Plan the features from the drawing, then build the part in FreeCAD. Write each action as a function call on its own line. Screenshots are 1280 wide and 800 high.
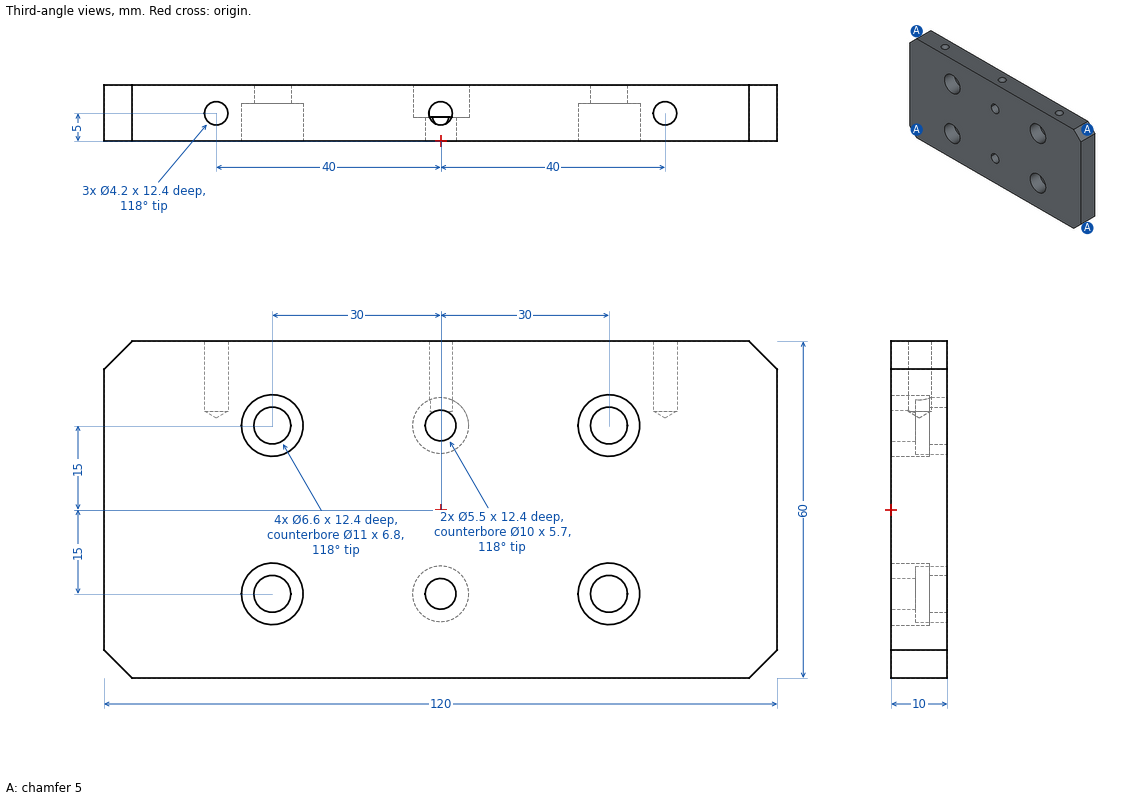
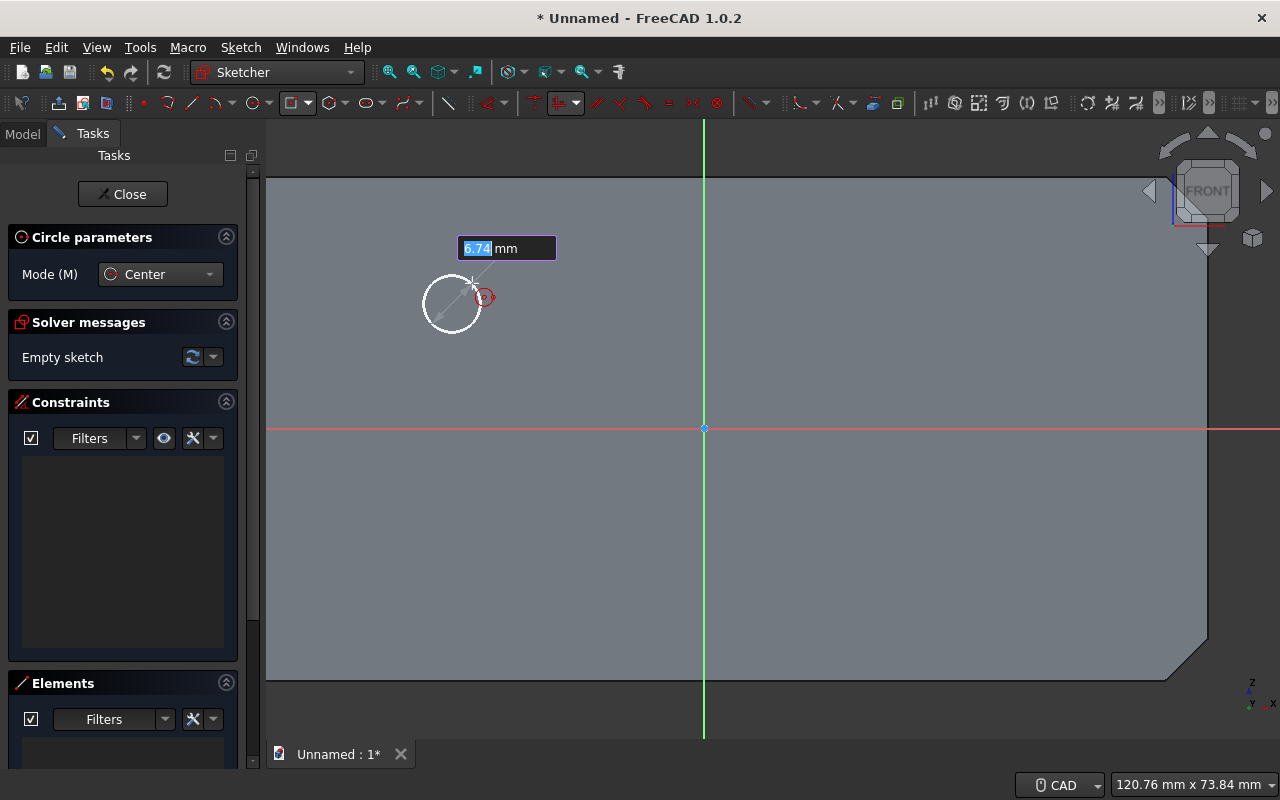
text(6.6)
key(Return)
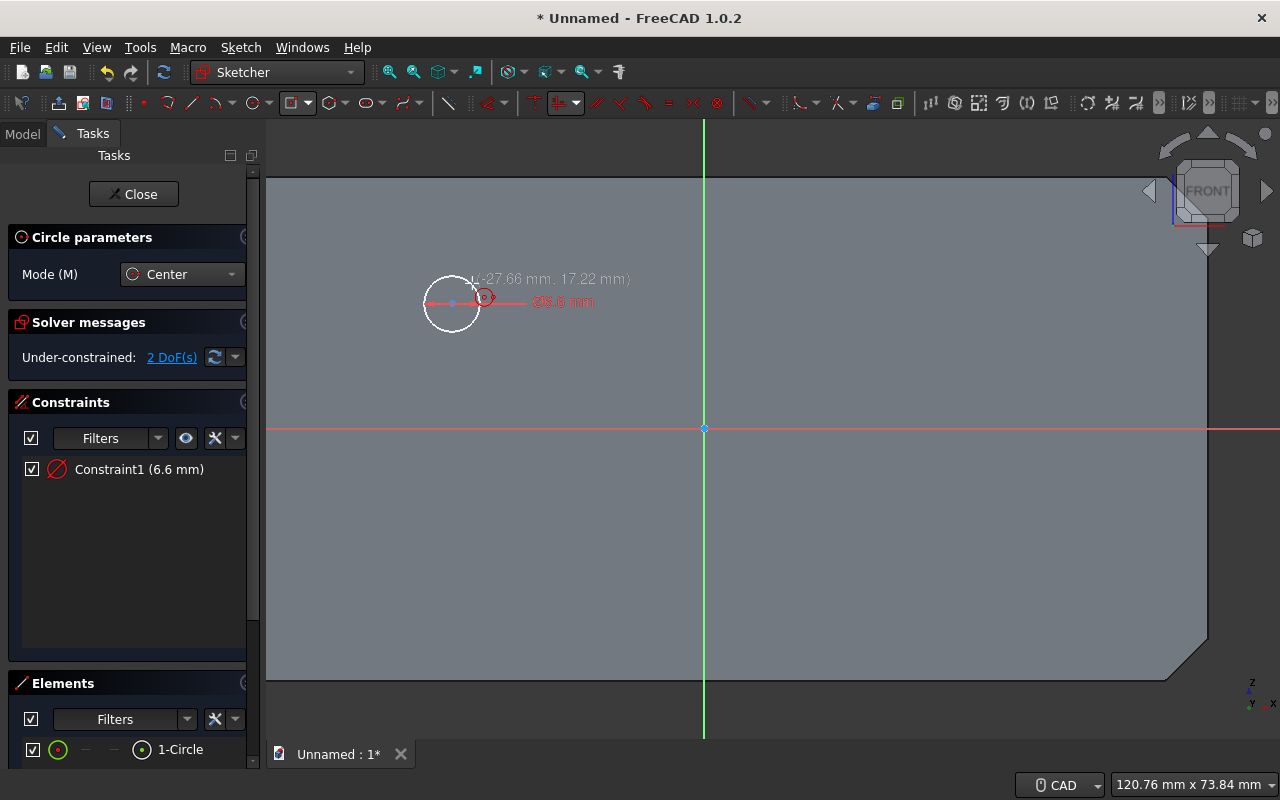
click(452, 555)
move(472, 535)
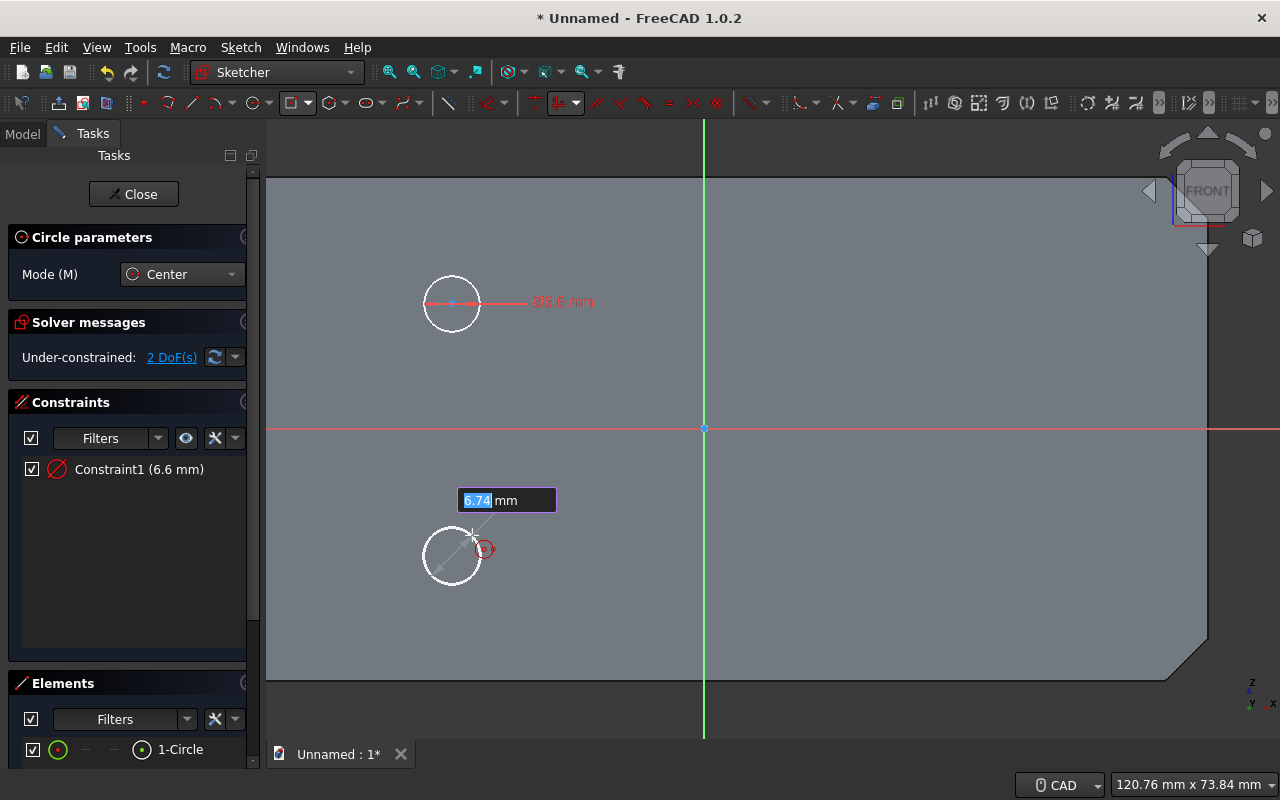
text(6.6)
key(Return)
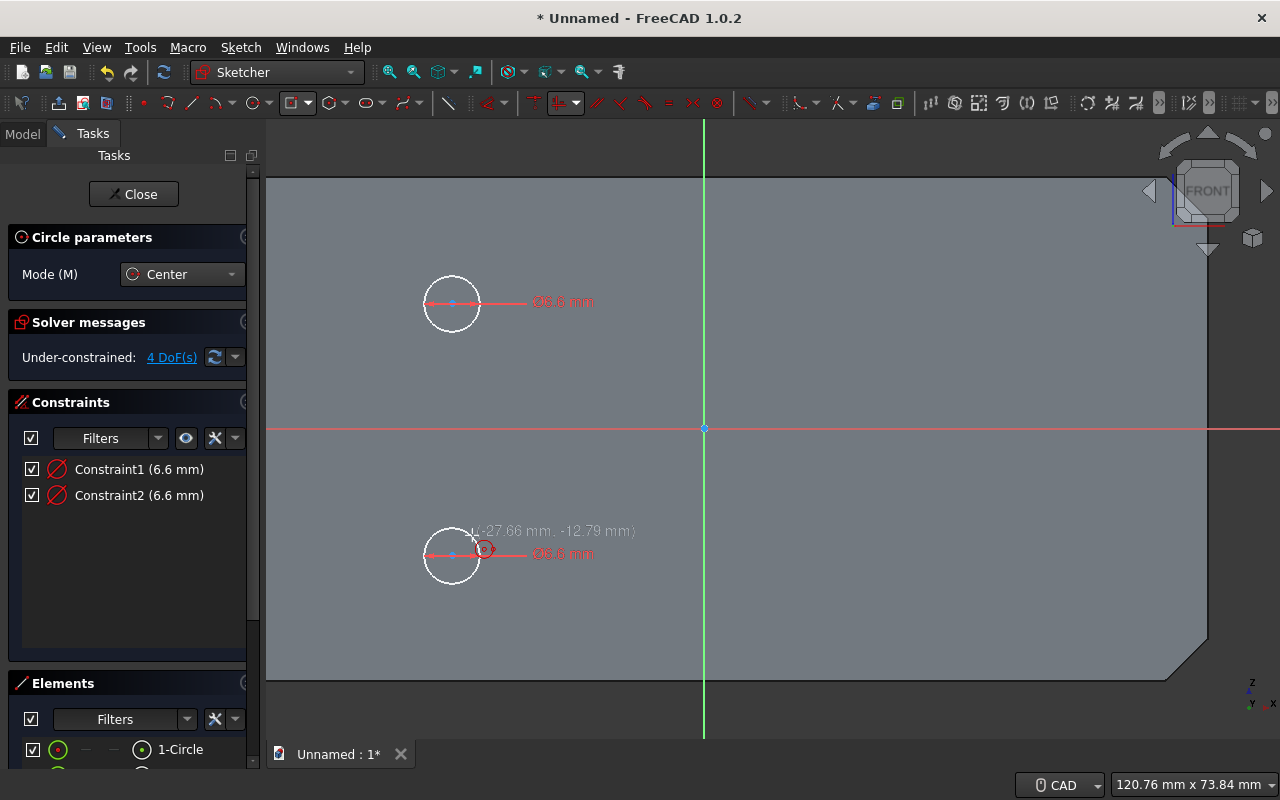
click(956, 303)
move(976, 283)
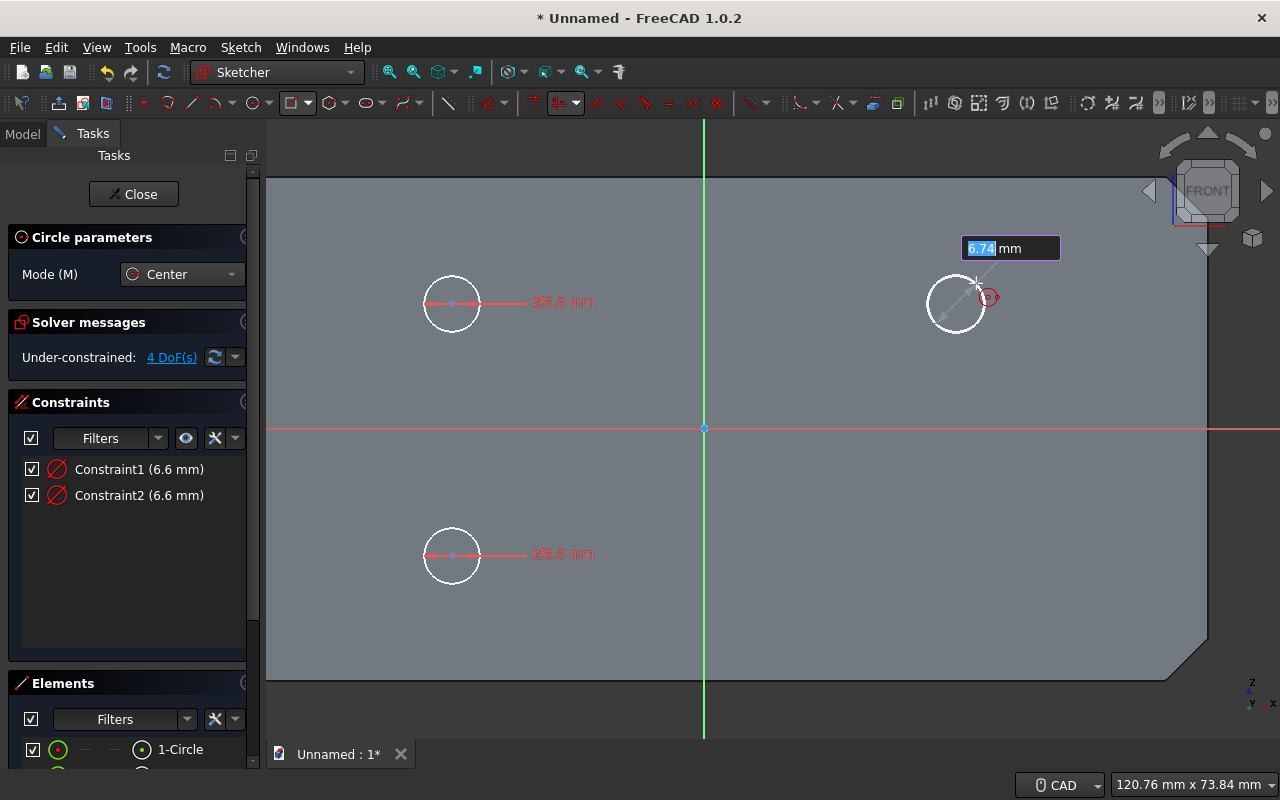
text(6.6)
key(Return)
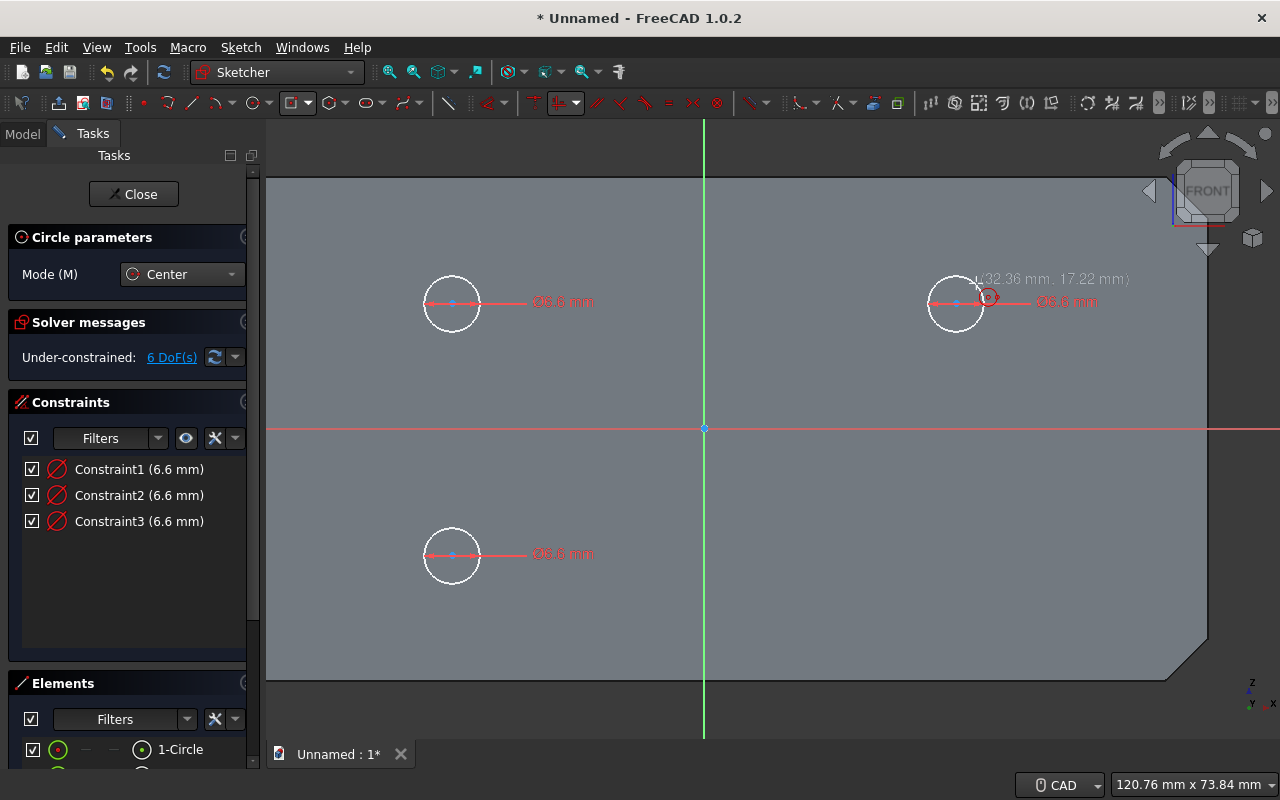
click(956, 555)
move(976, 535)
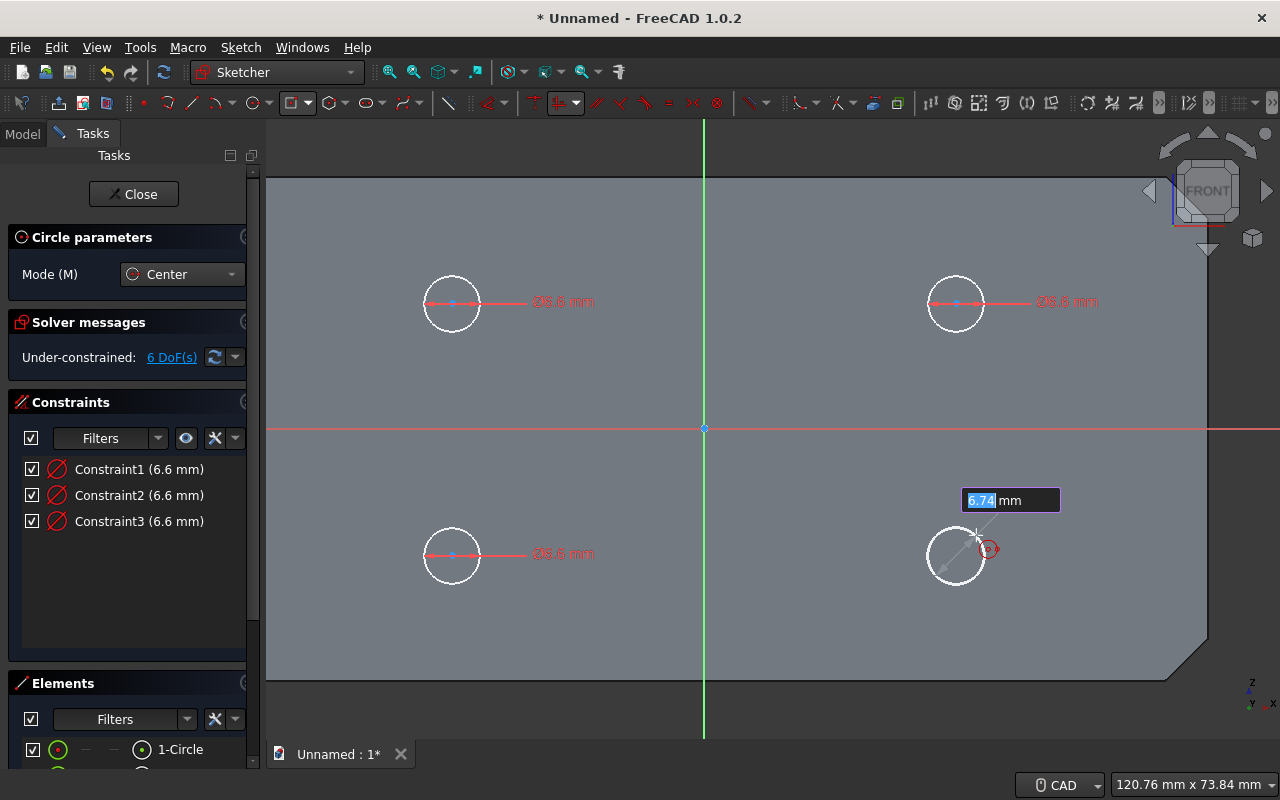
text(6.6)
key(Return)
key(Escape)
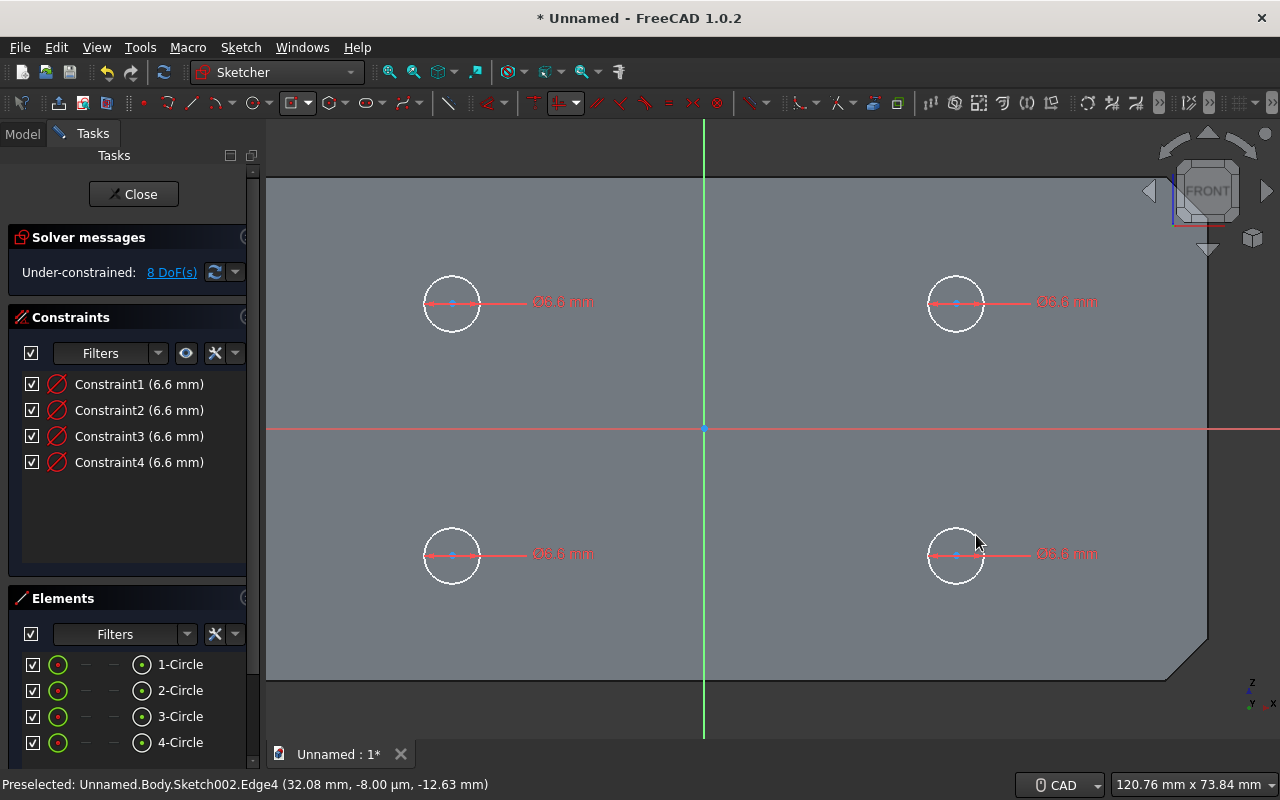
click(452, 304)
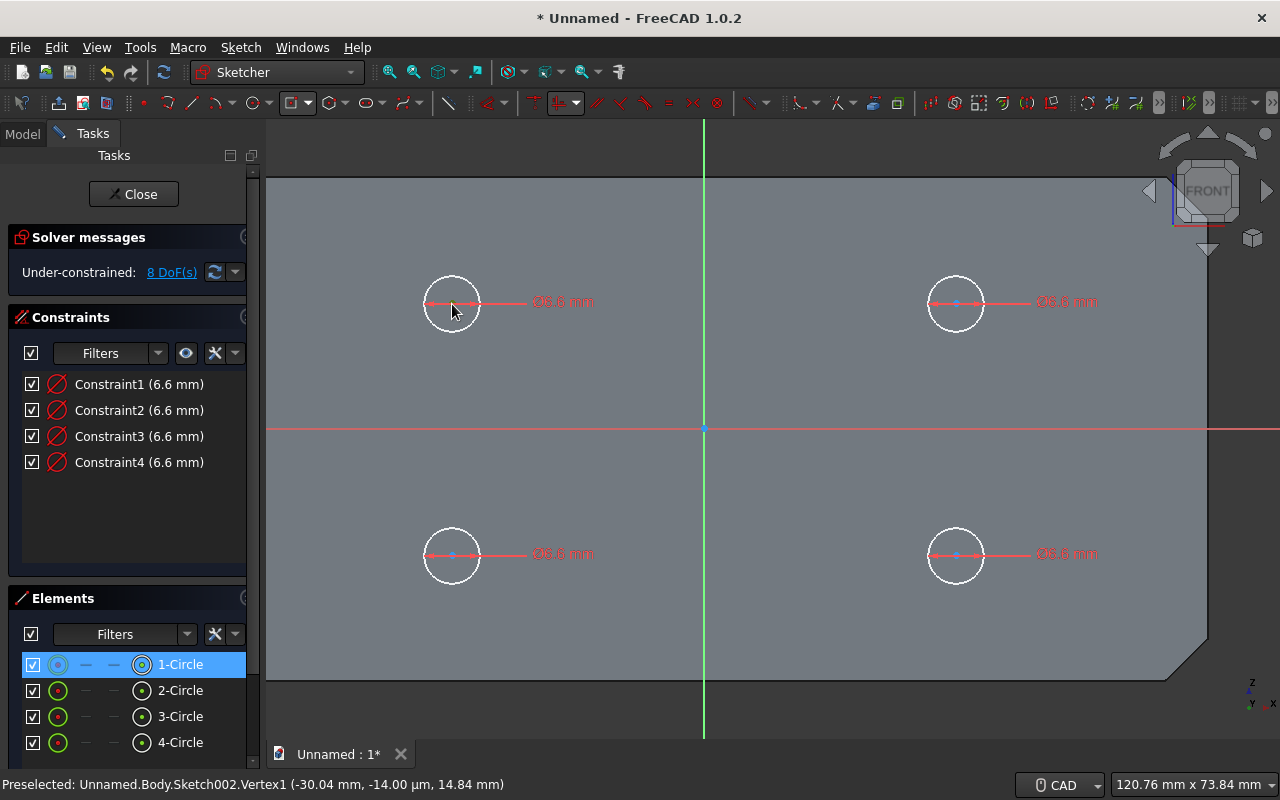
click(452, 556)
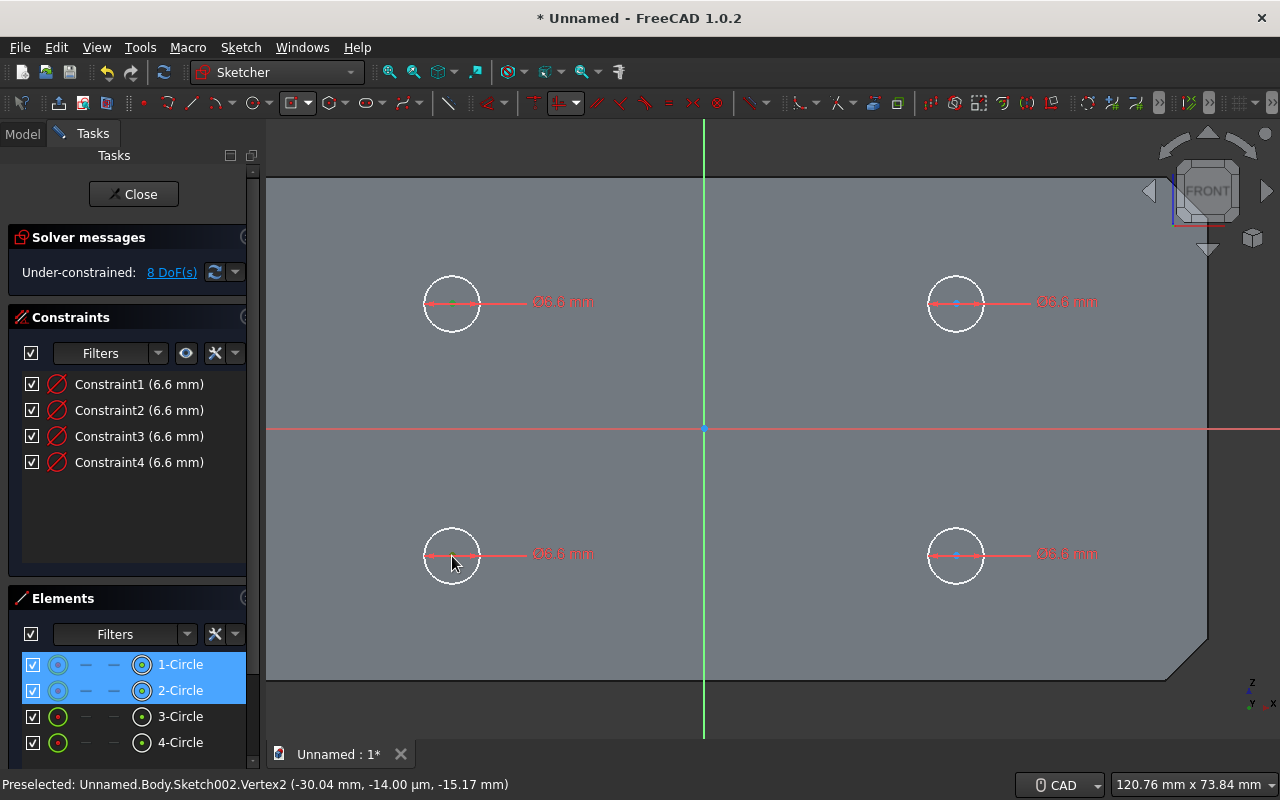
key(v)